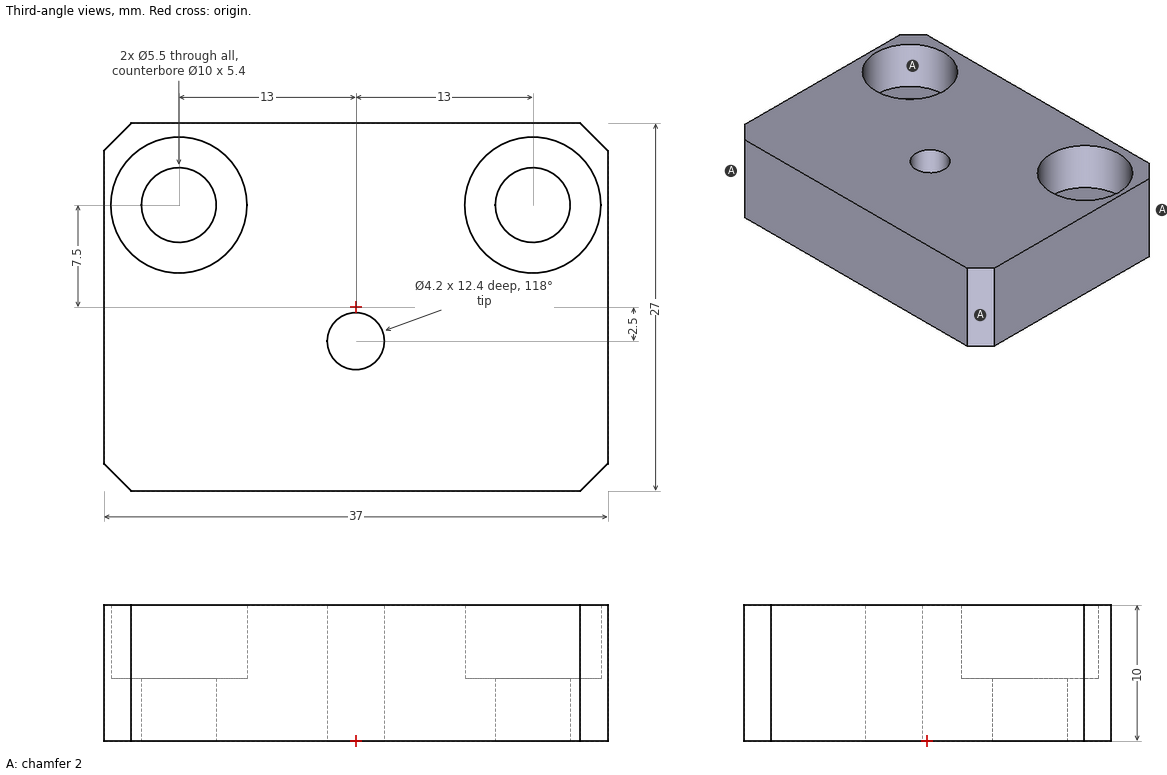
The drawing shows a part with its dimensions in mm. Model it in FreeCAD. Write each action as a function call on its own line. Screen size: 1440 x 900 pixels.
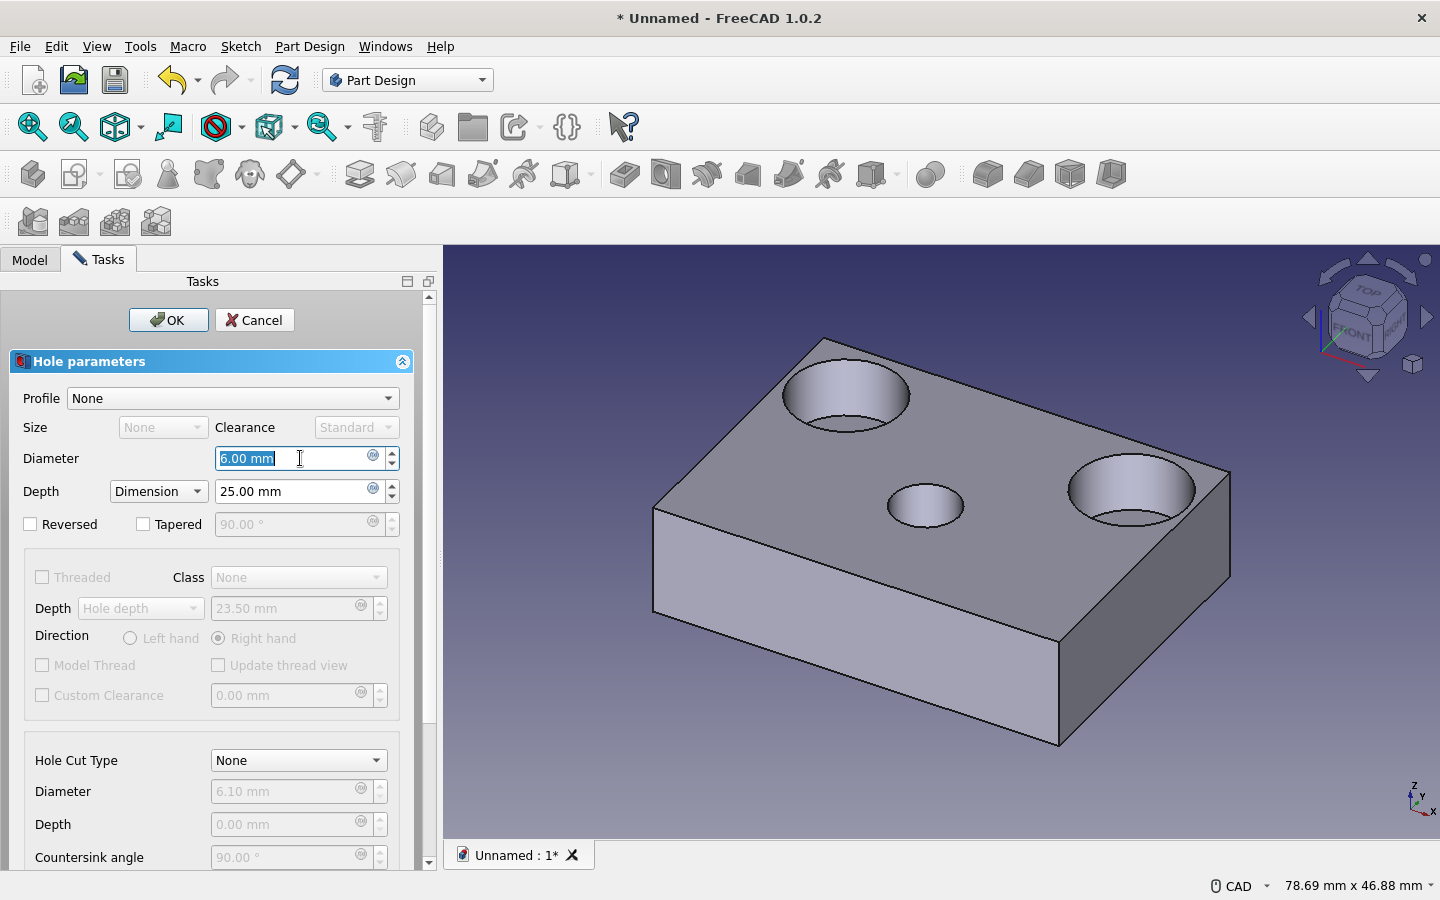
text(4.2)
key(Tab)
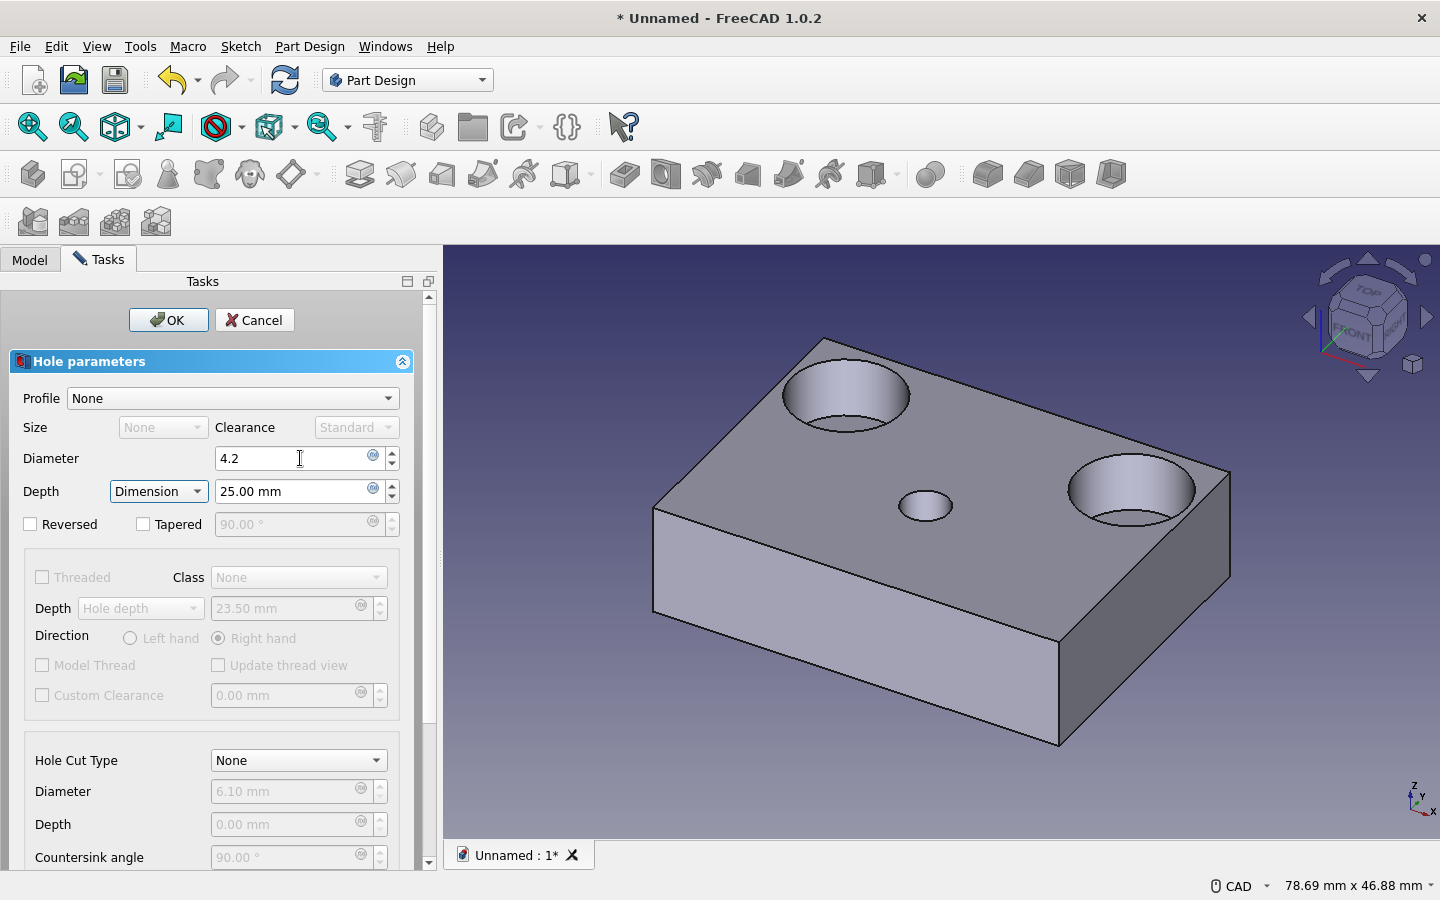
triple_click(300, 492)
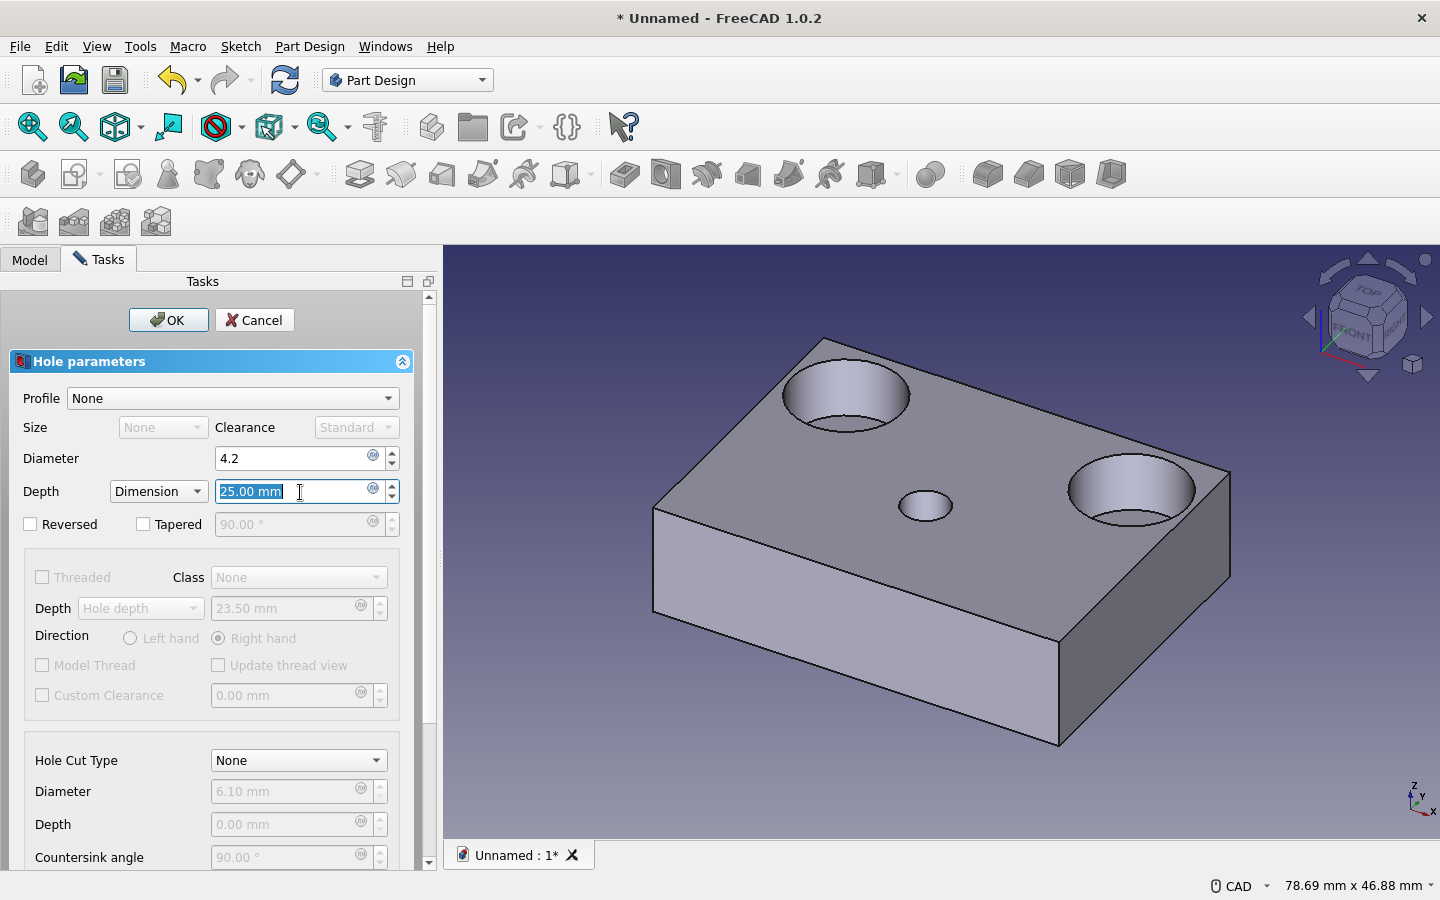
text(12.4)
key(Tab)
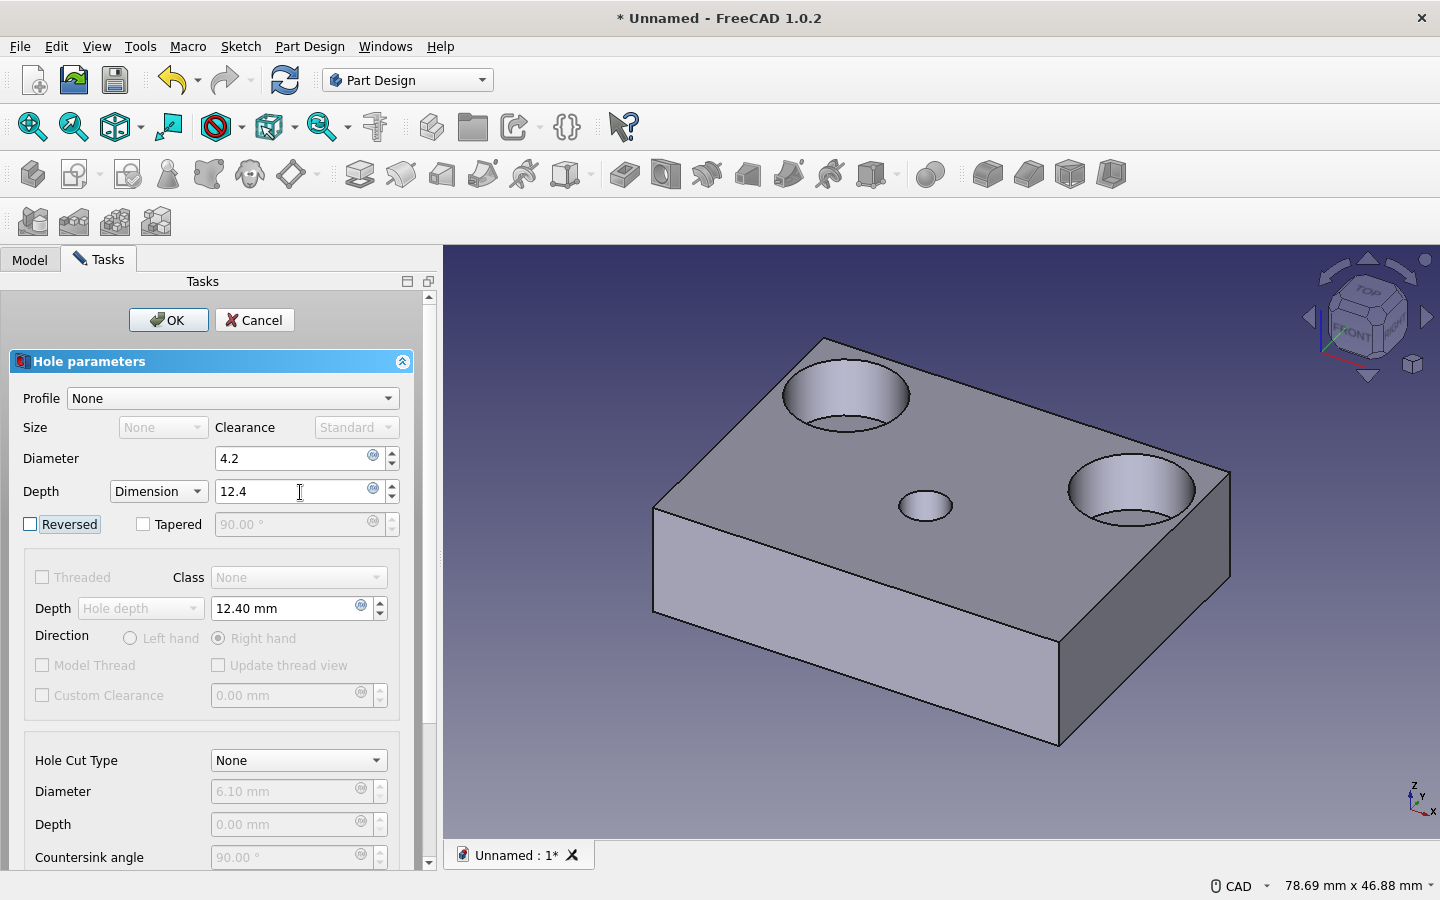
click(169, 320)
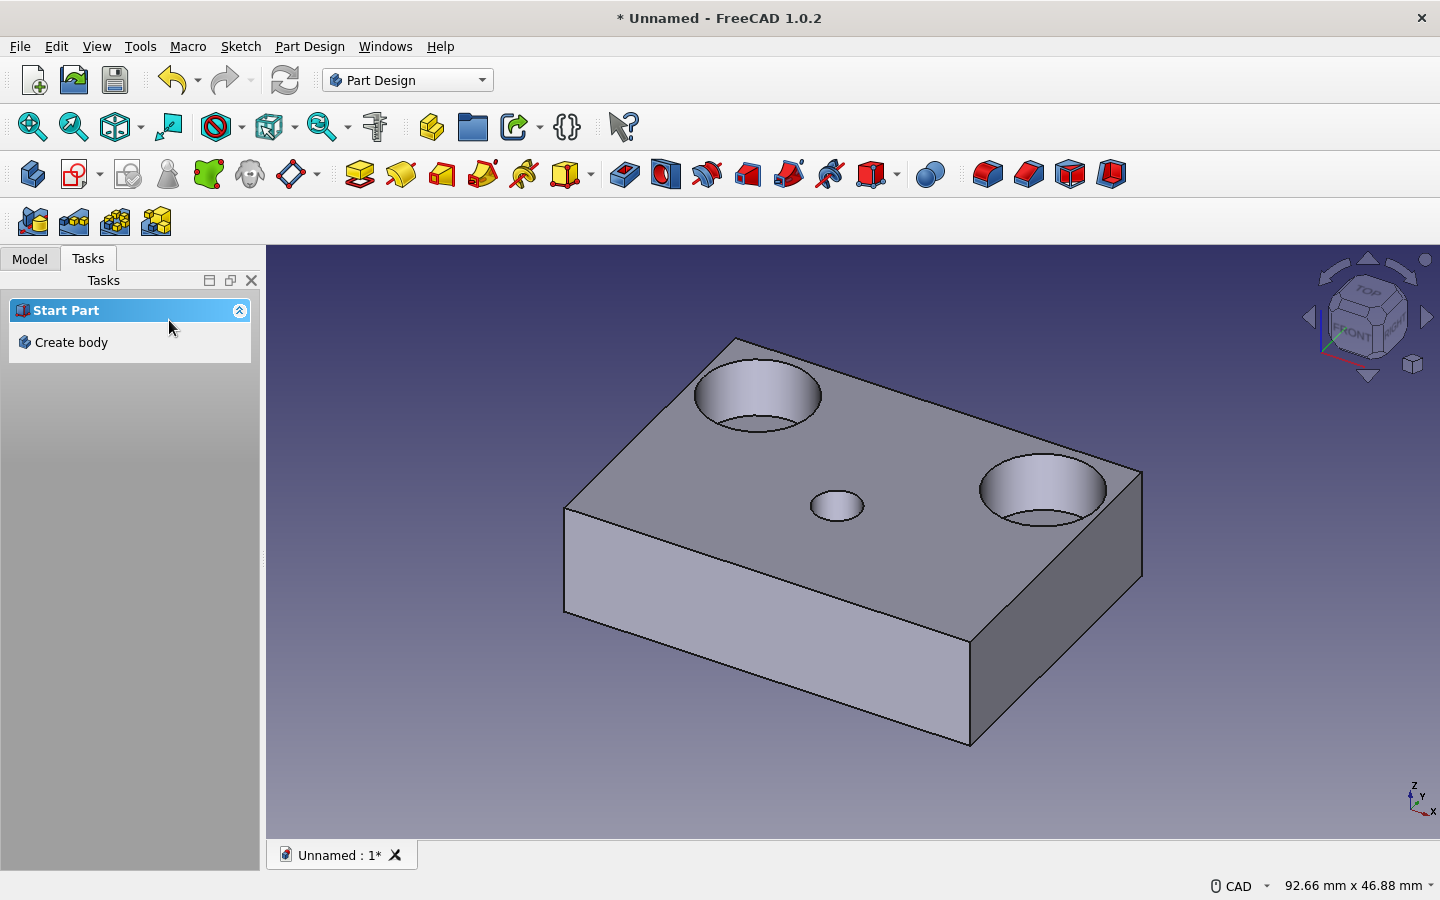
click(970, 693)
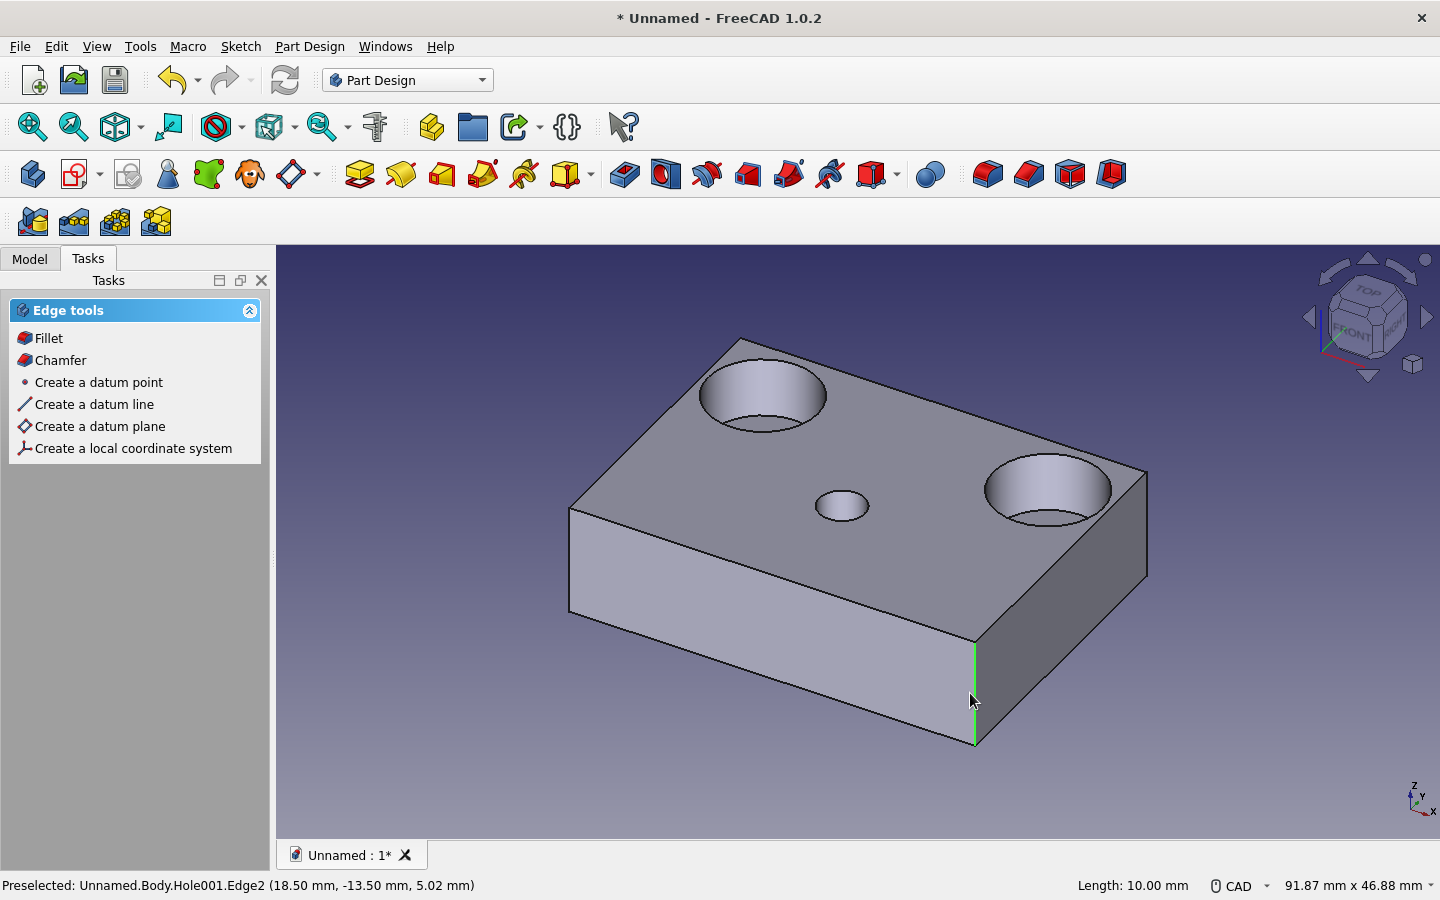
key(0)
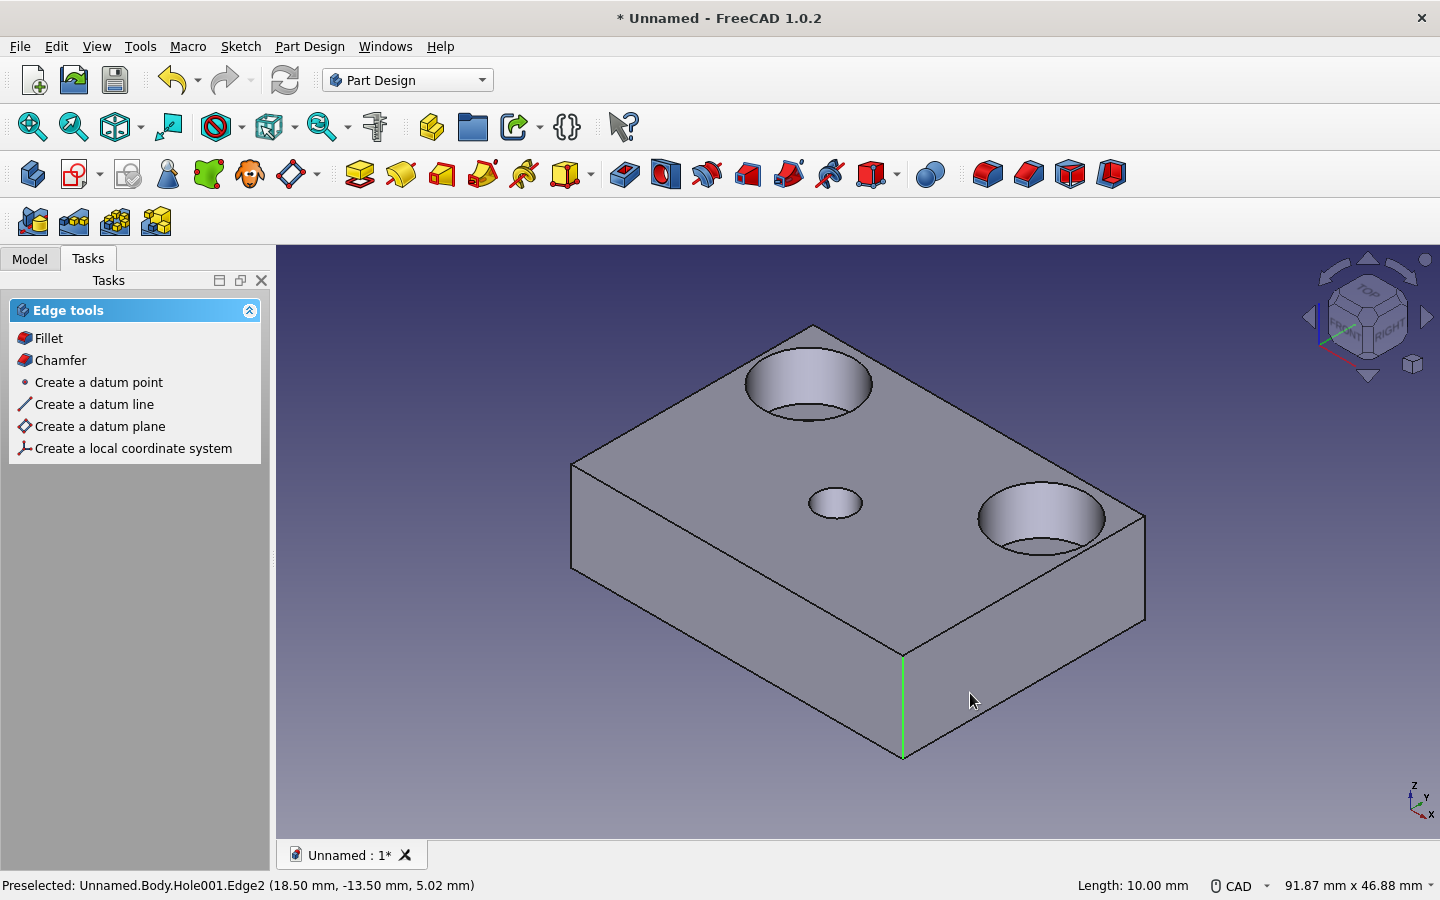
key(2)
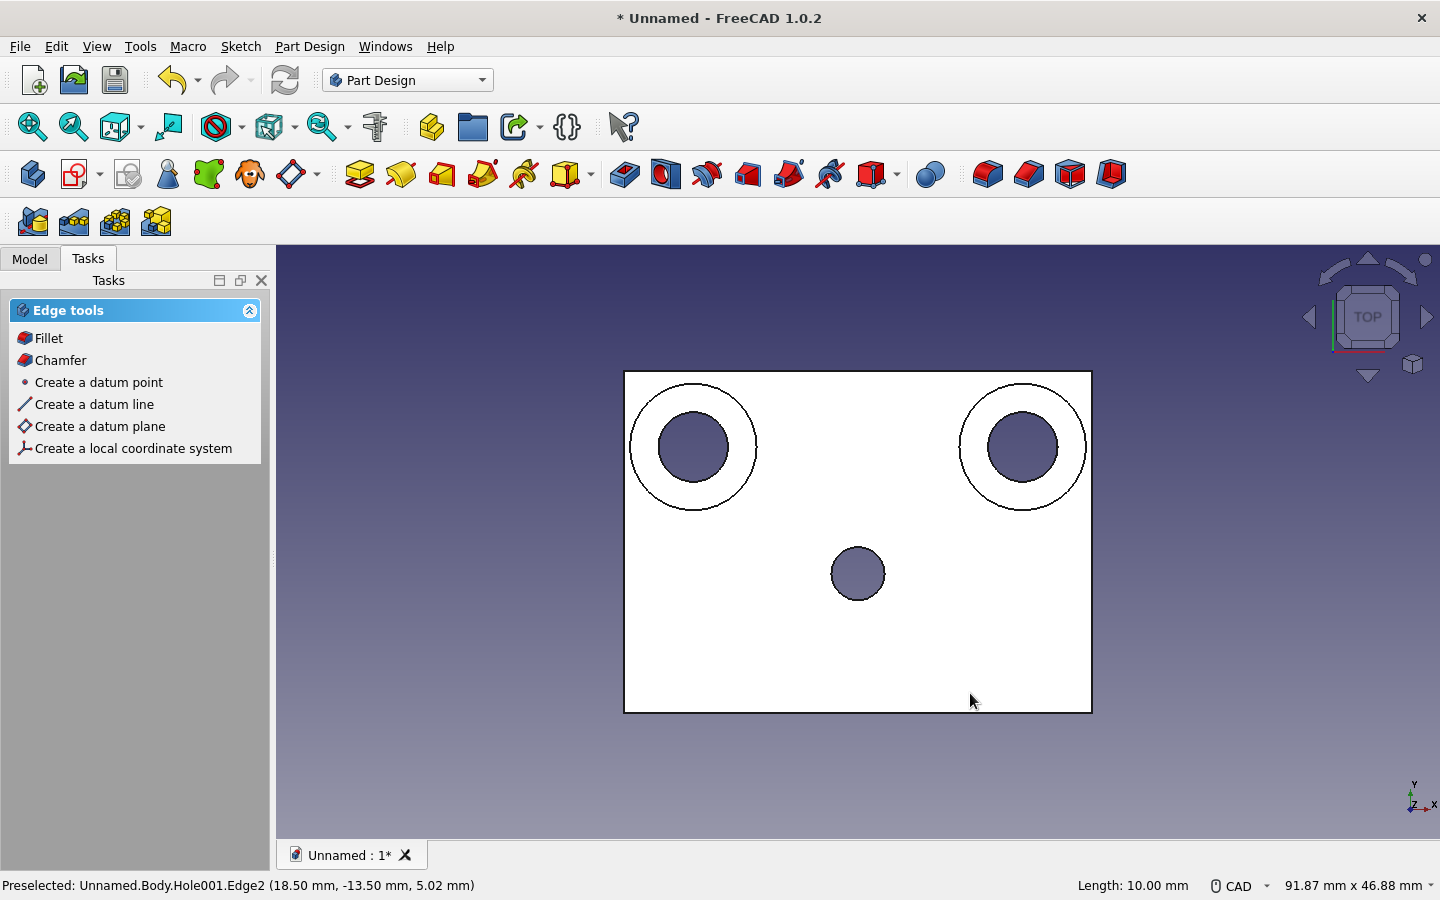
key(1)